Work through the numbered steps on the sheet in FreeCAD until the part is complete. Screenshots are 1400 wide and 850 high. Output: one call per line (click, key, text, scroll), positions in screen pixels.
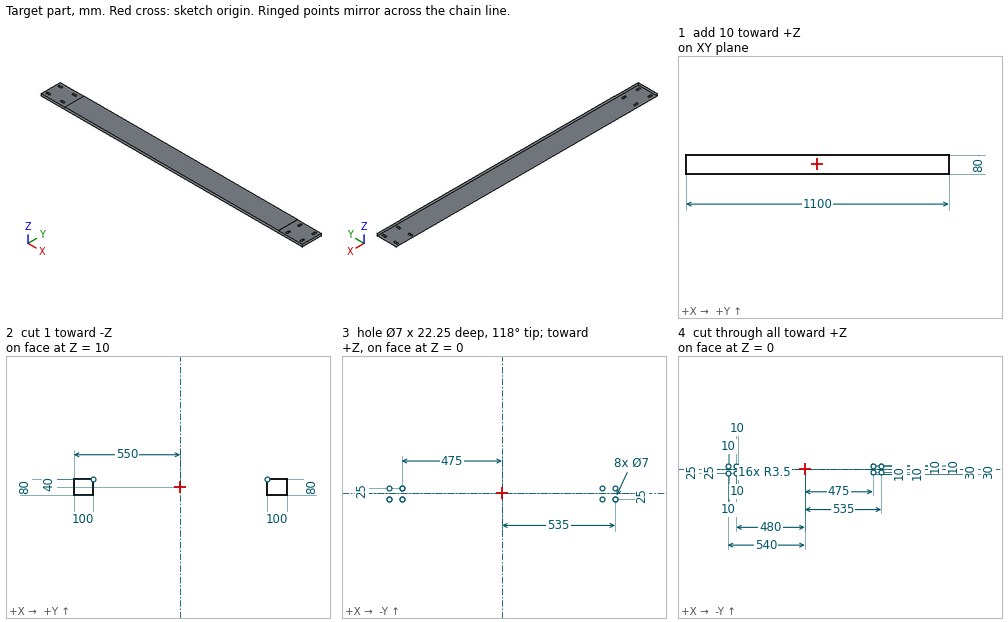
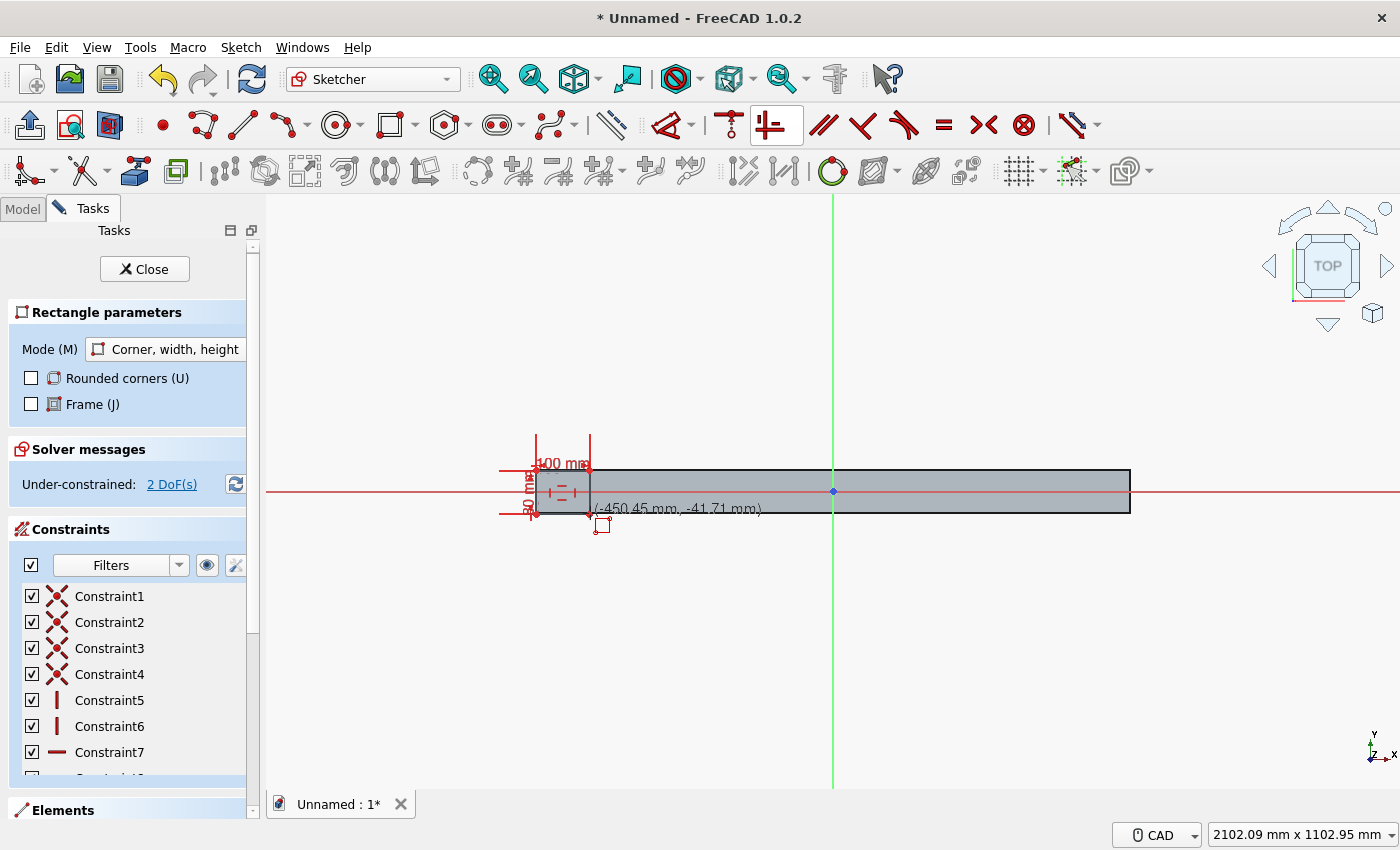
click(1076, 470)
move(1130, 513)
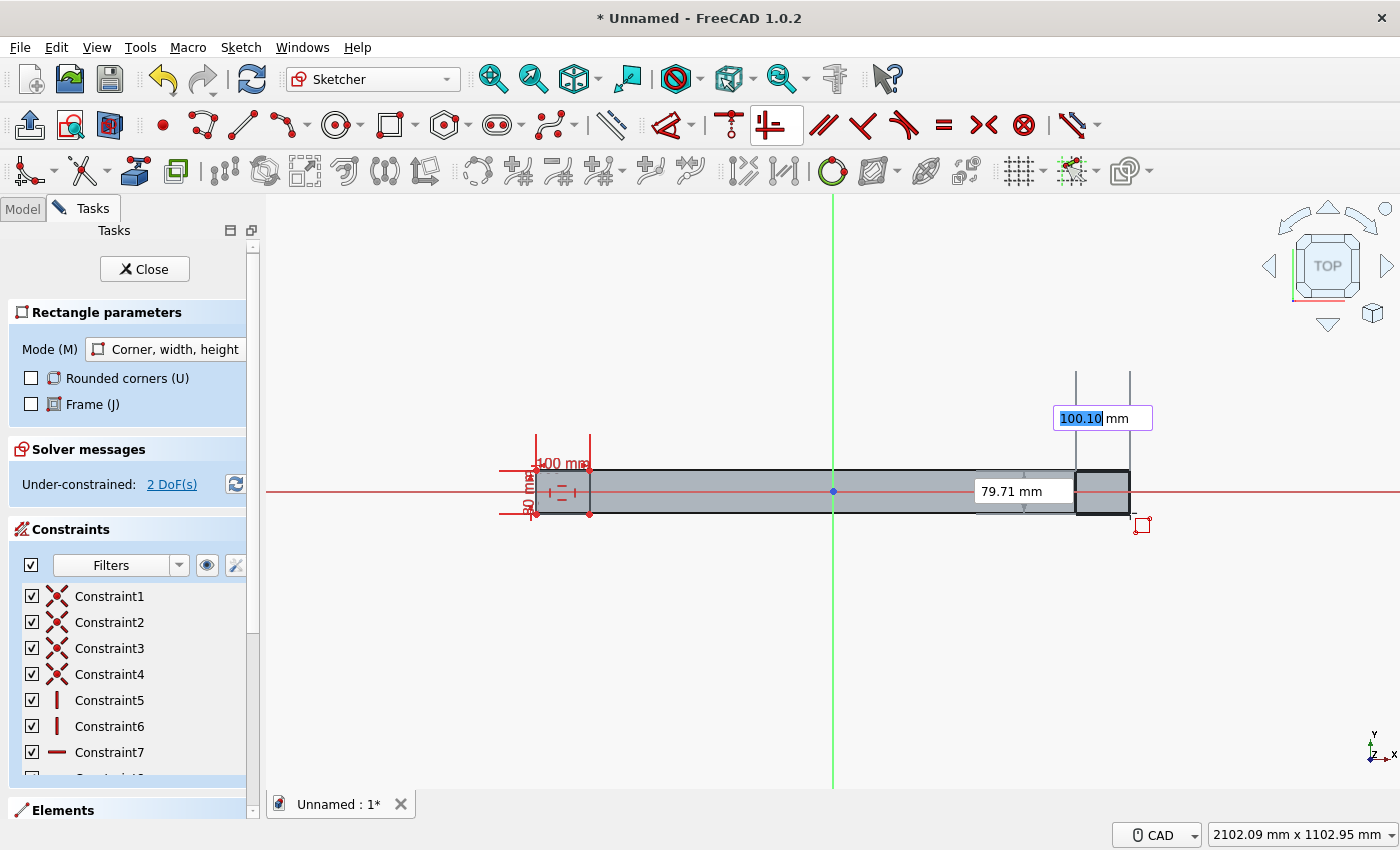
text(100)
key(Tab)
text(80)
key(Return)
key(Escape)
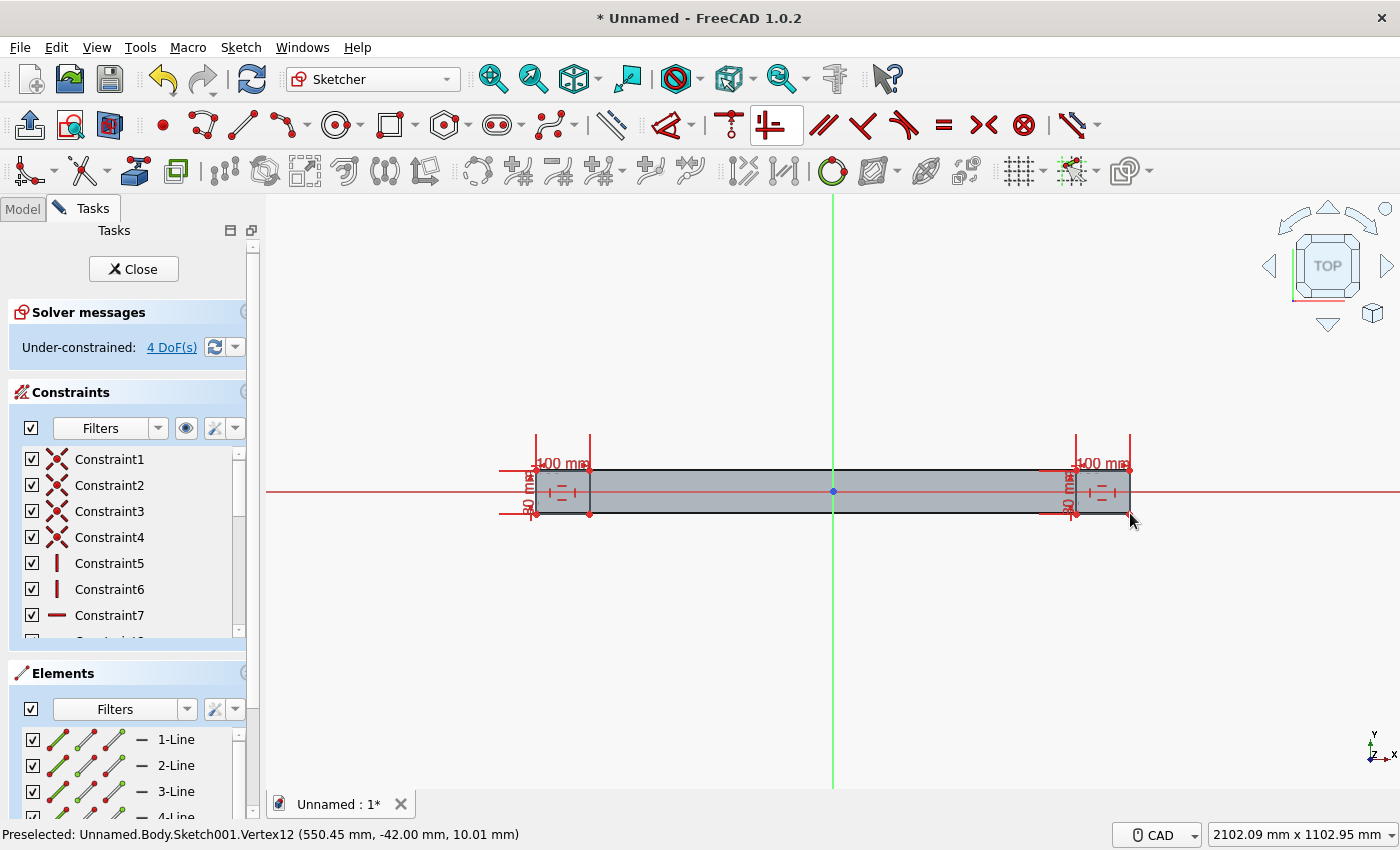
click(590, 471)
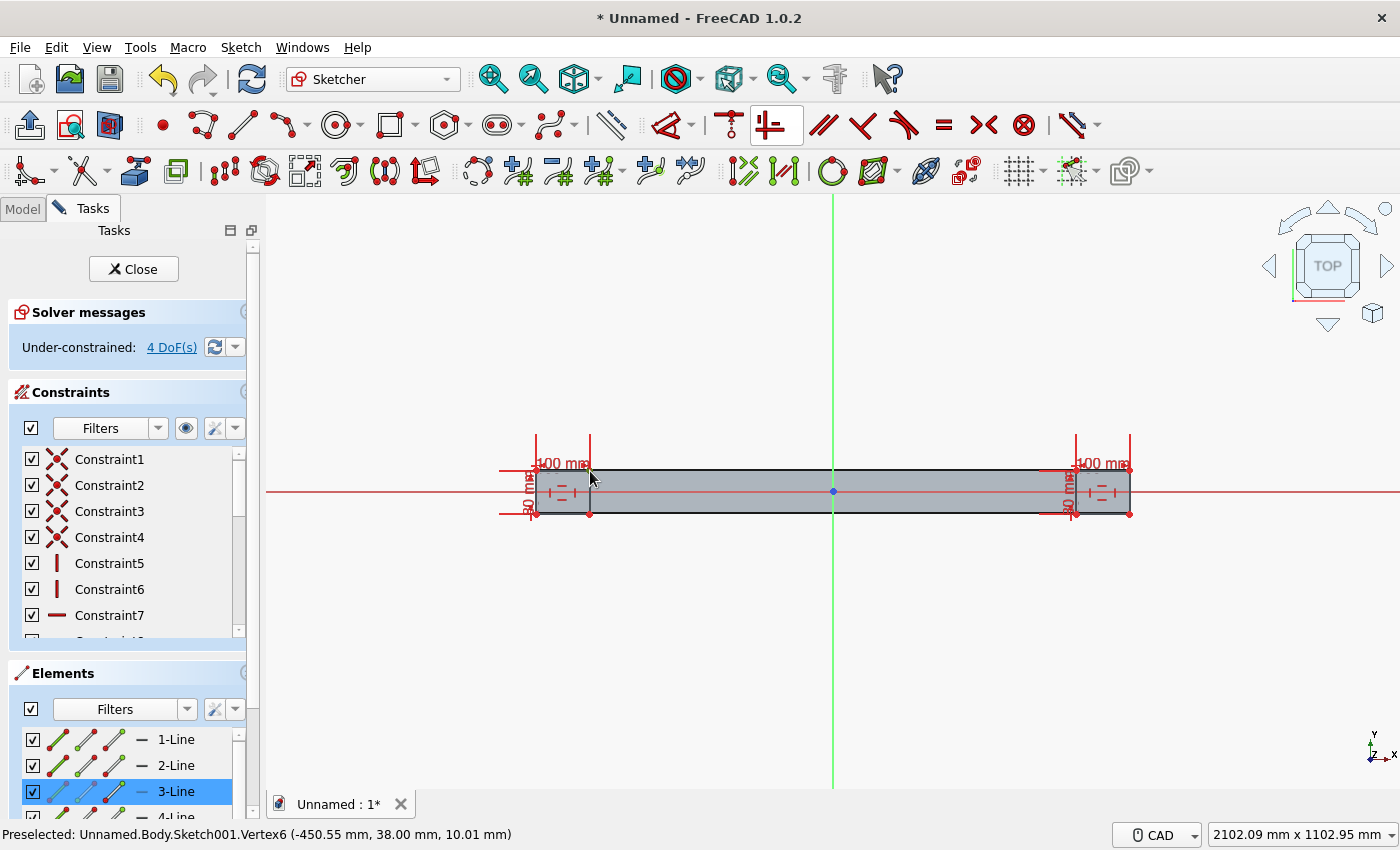
click(1076, 471)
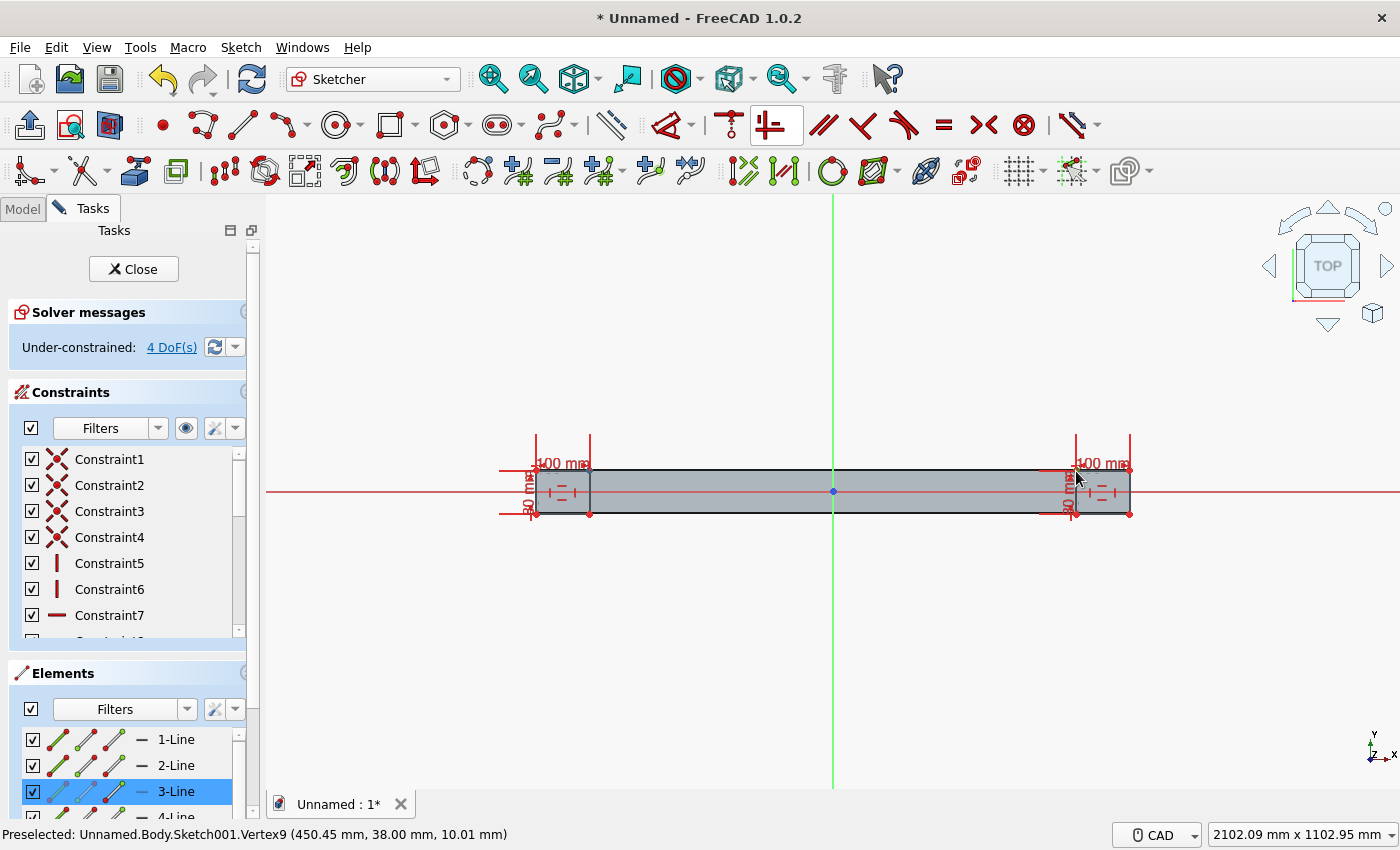
click(833, 722)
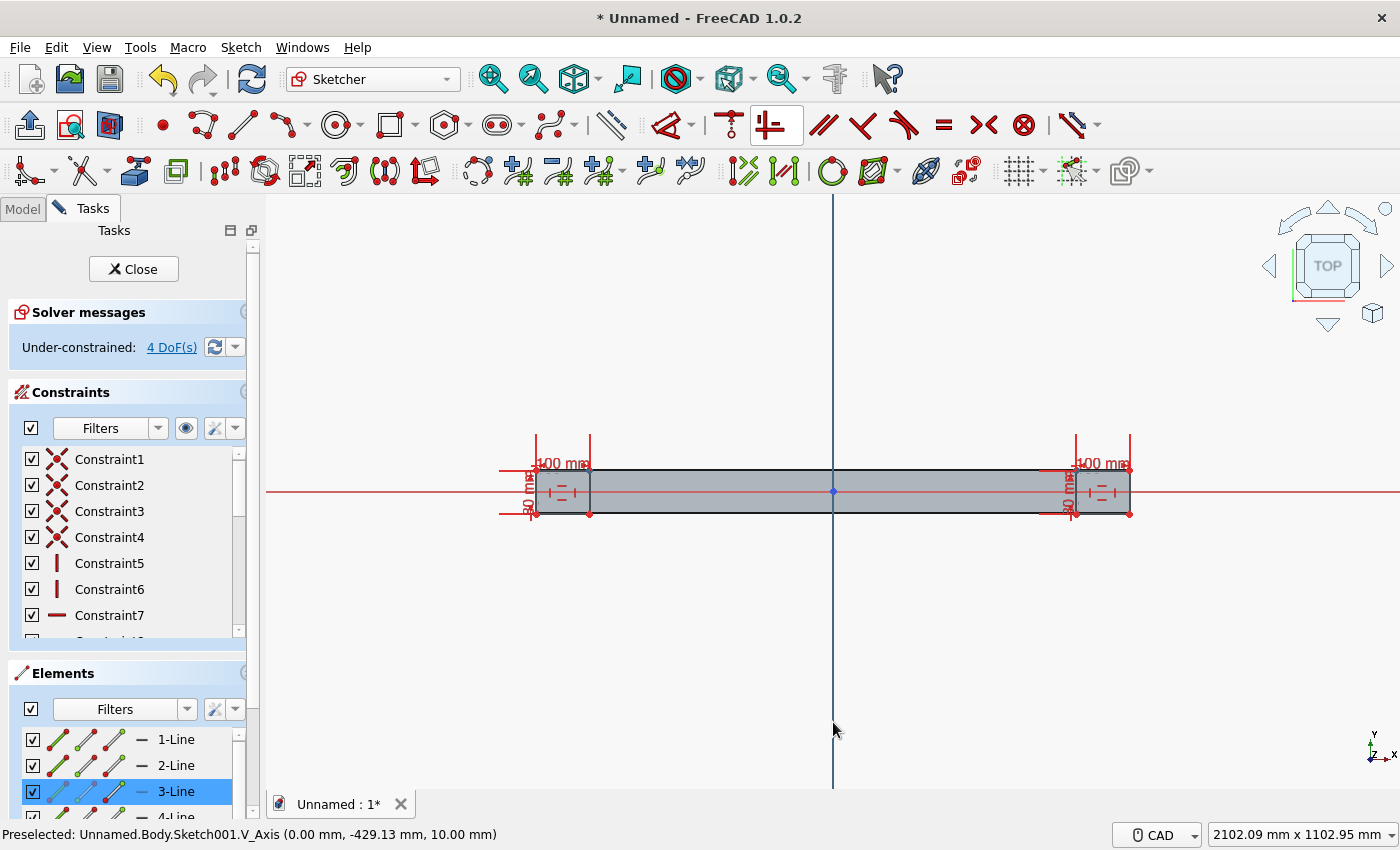
key(s)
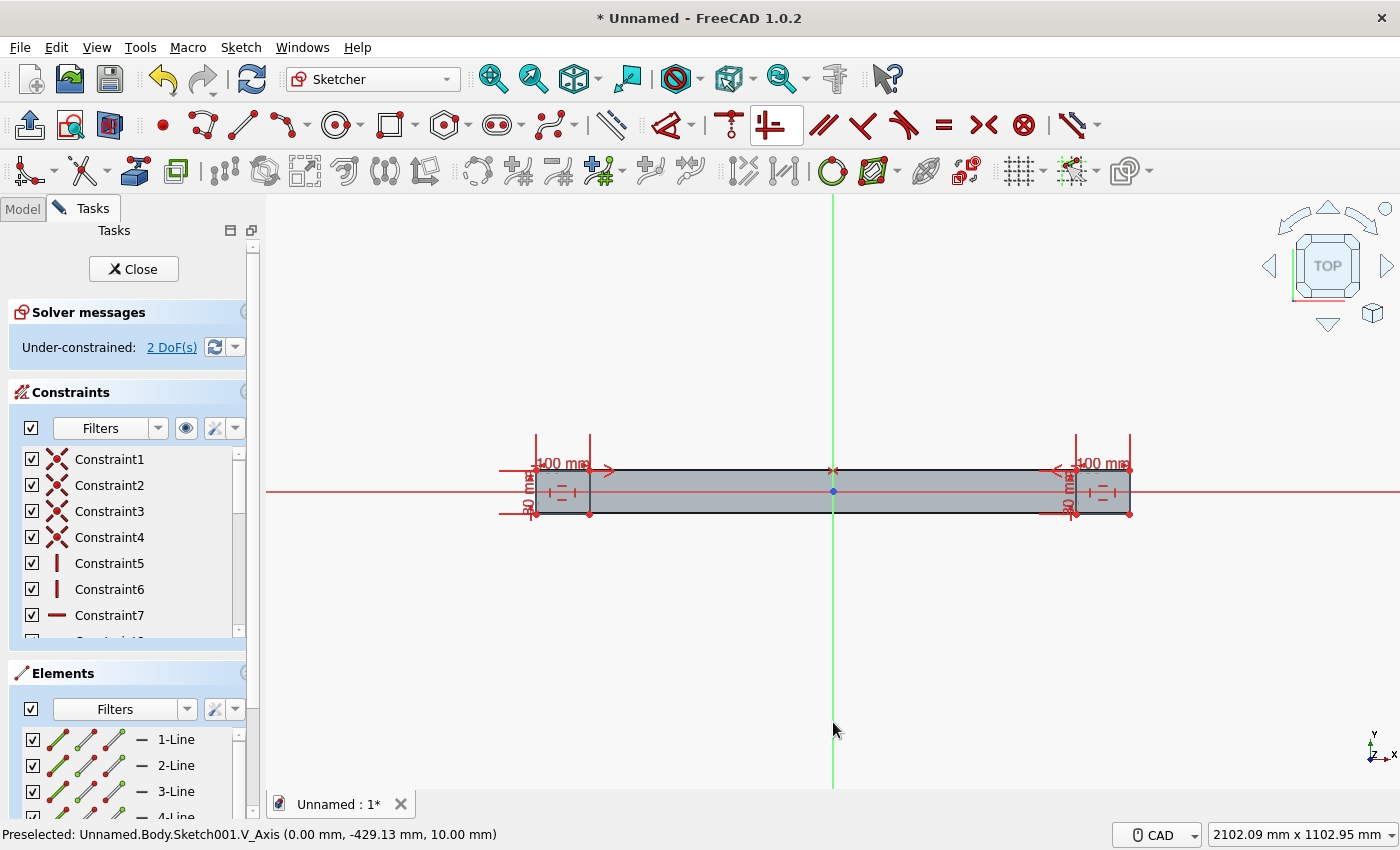
click(666, 126)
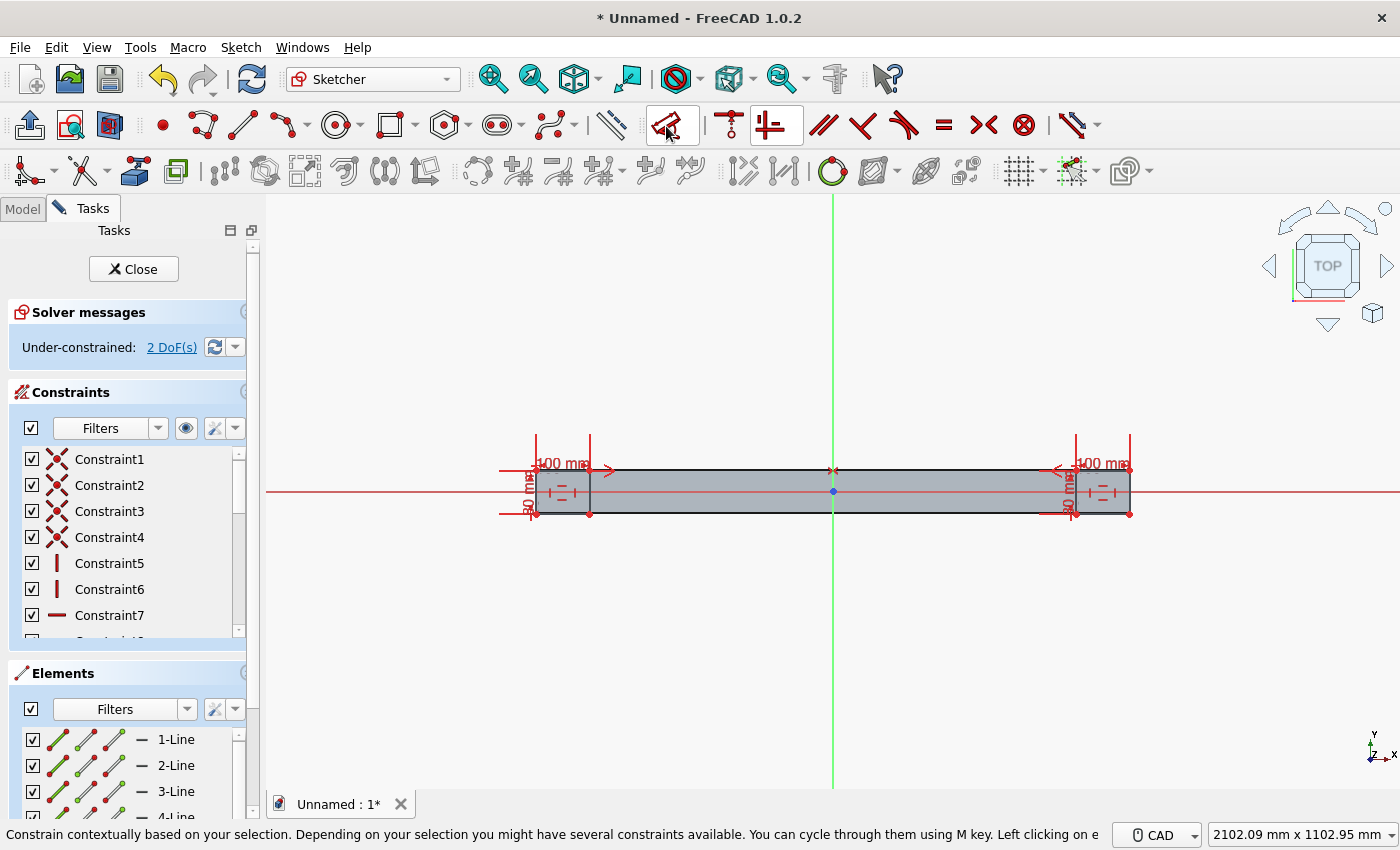
scroll(536, 471, up, 4)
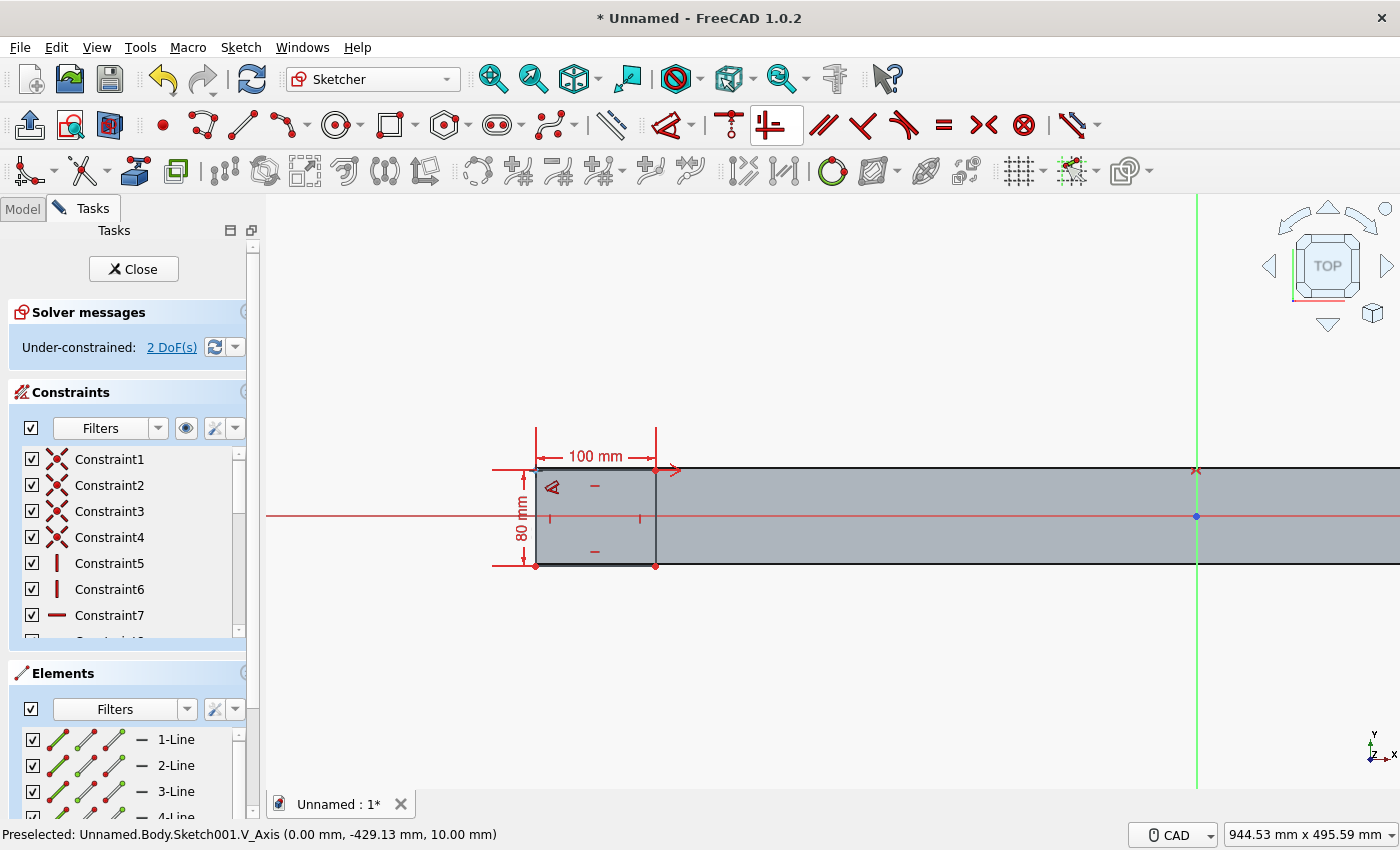
click(536, 470)
click(502, 493)